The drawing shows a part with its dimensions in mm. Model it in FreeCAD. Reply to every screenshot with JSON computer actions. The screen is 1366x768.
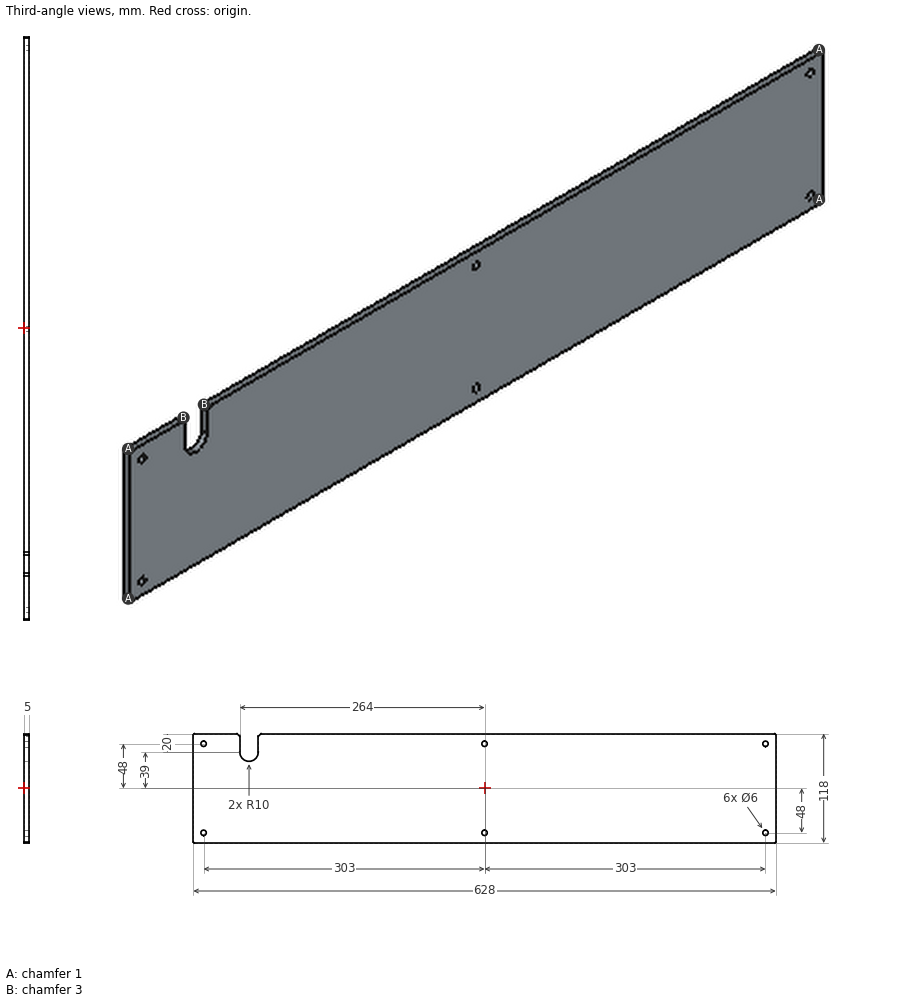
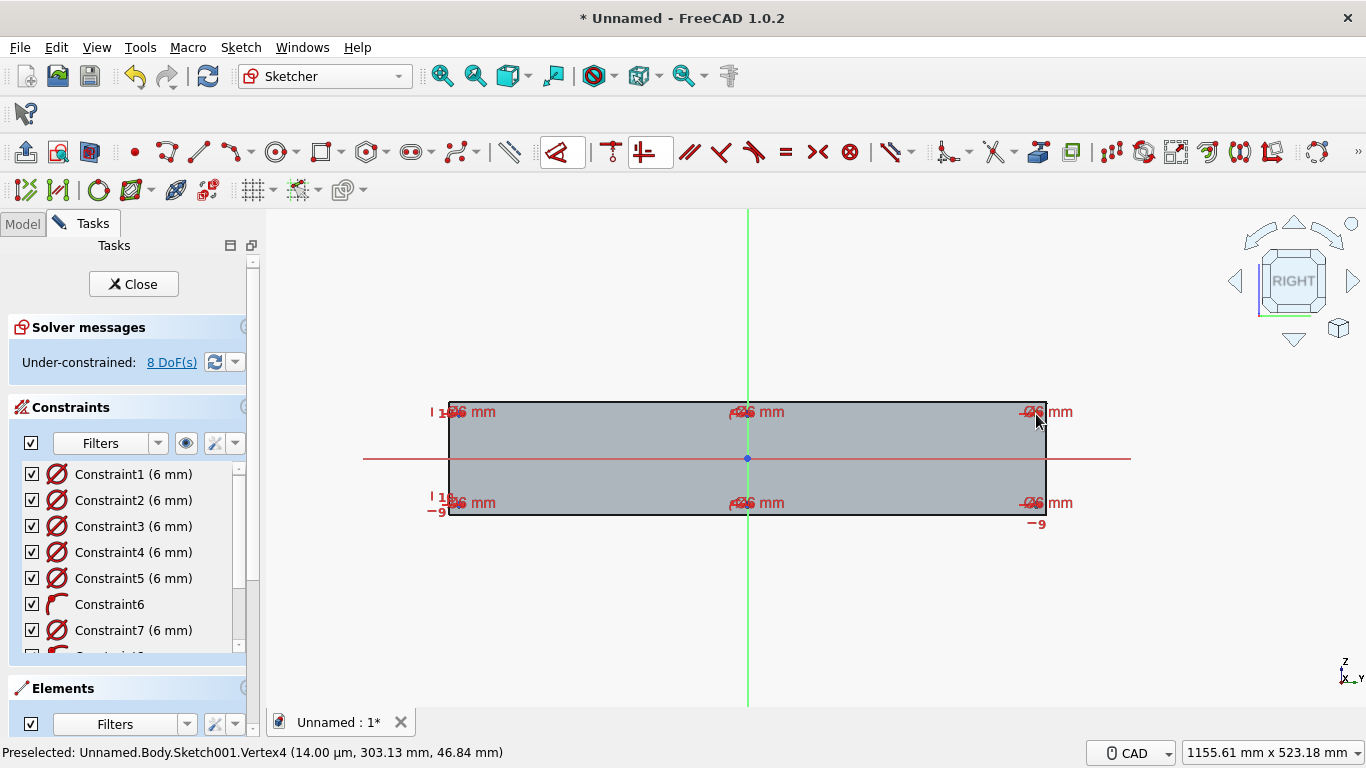
{"action": "left_click", "coordinate": [668, 152]}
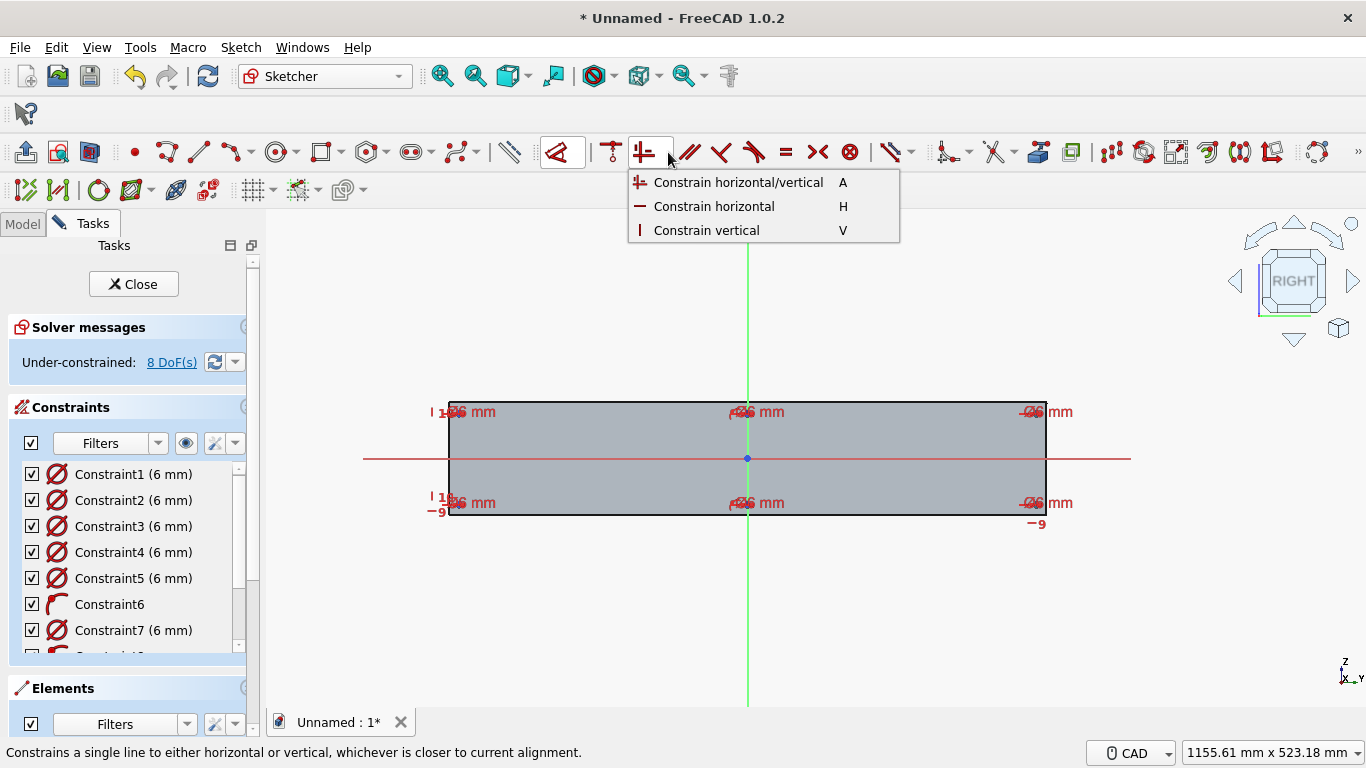
{"action": "left_click", "coordinate": [764, 230]}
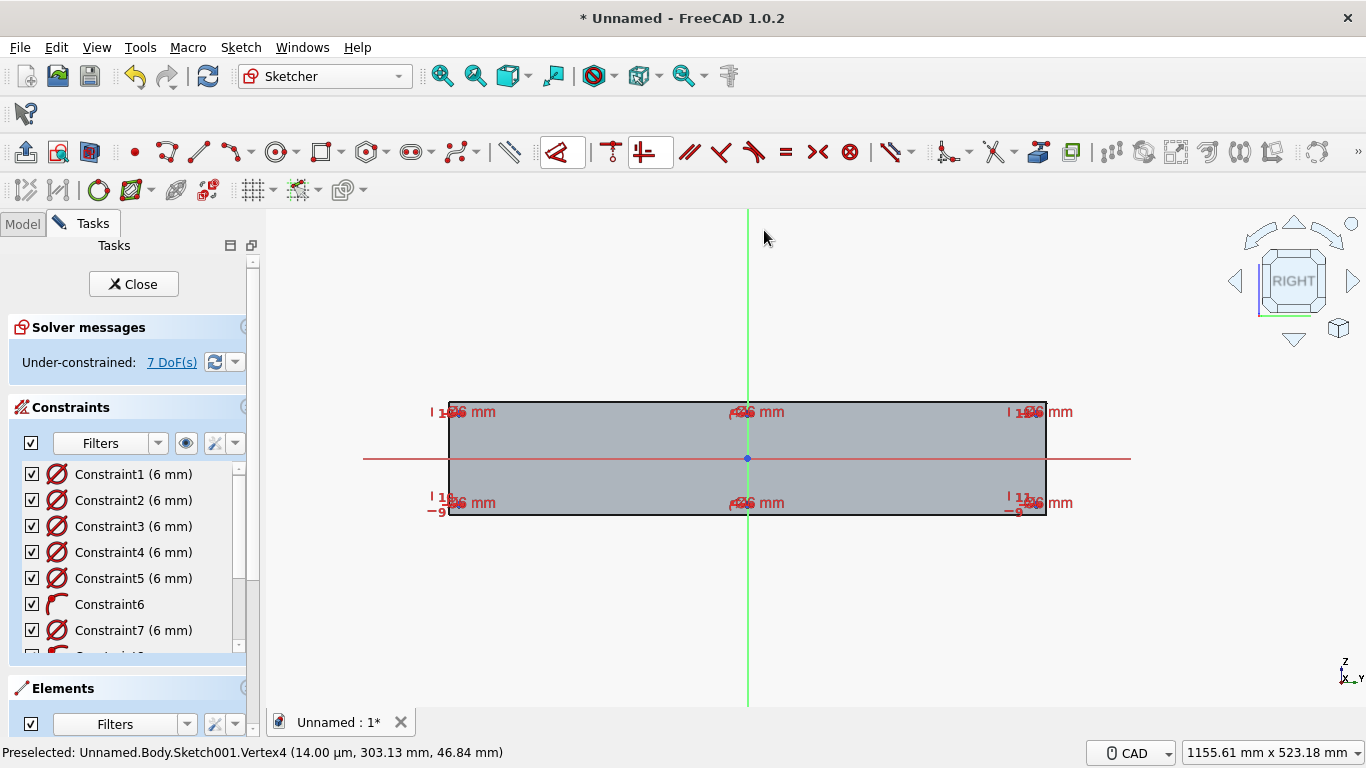
{"action": "left_click", "coordinate": [459, 414]}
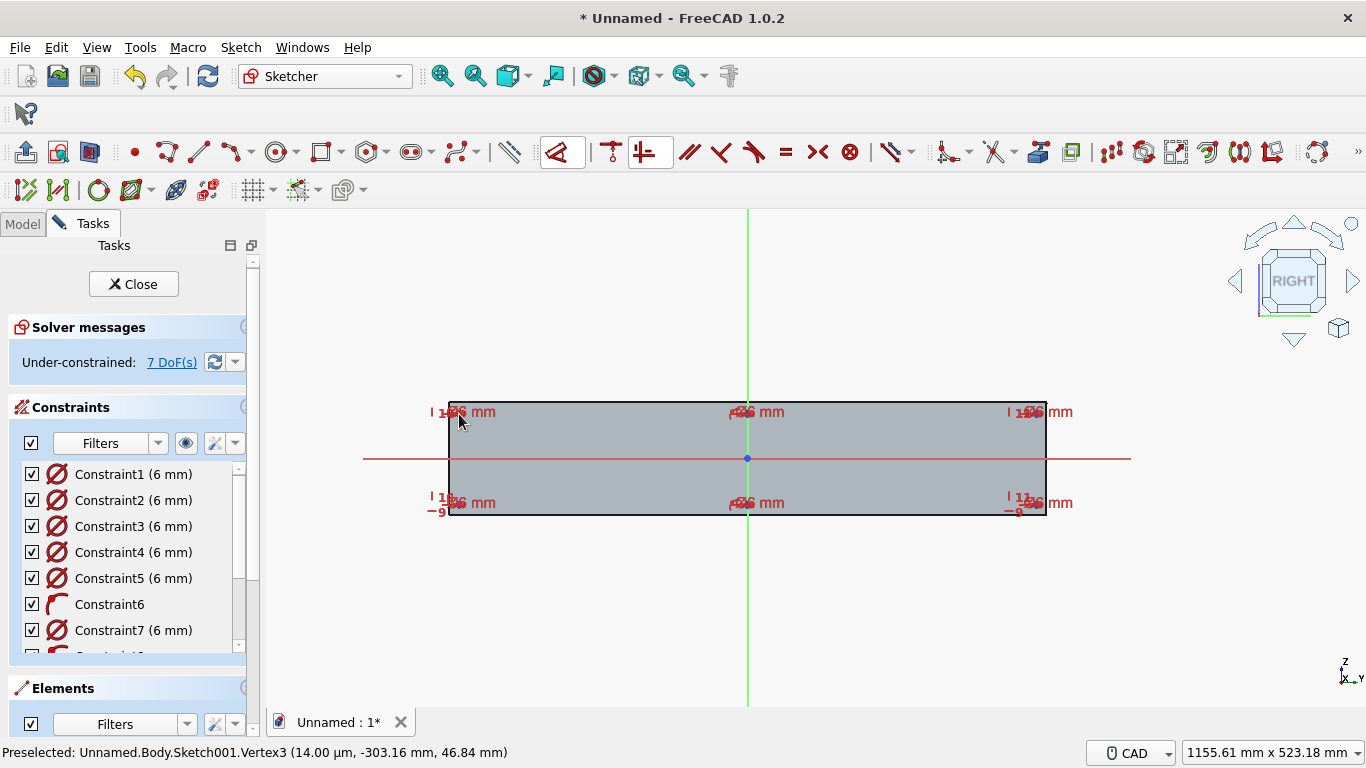
{"action": "left_click", "coordinate": [1036, 414]}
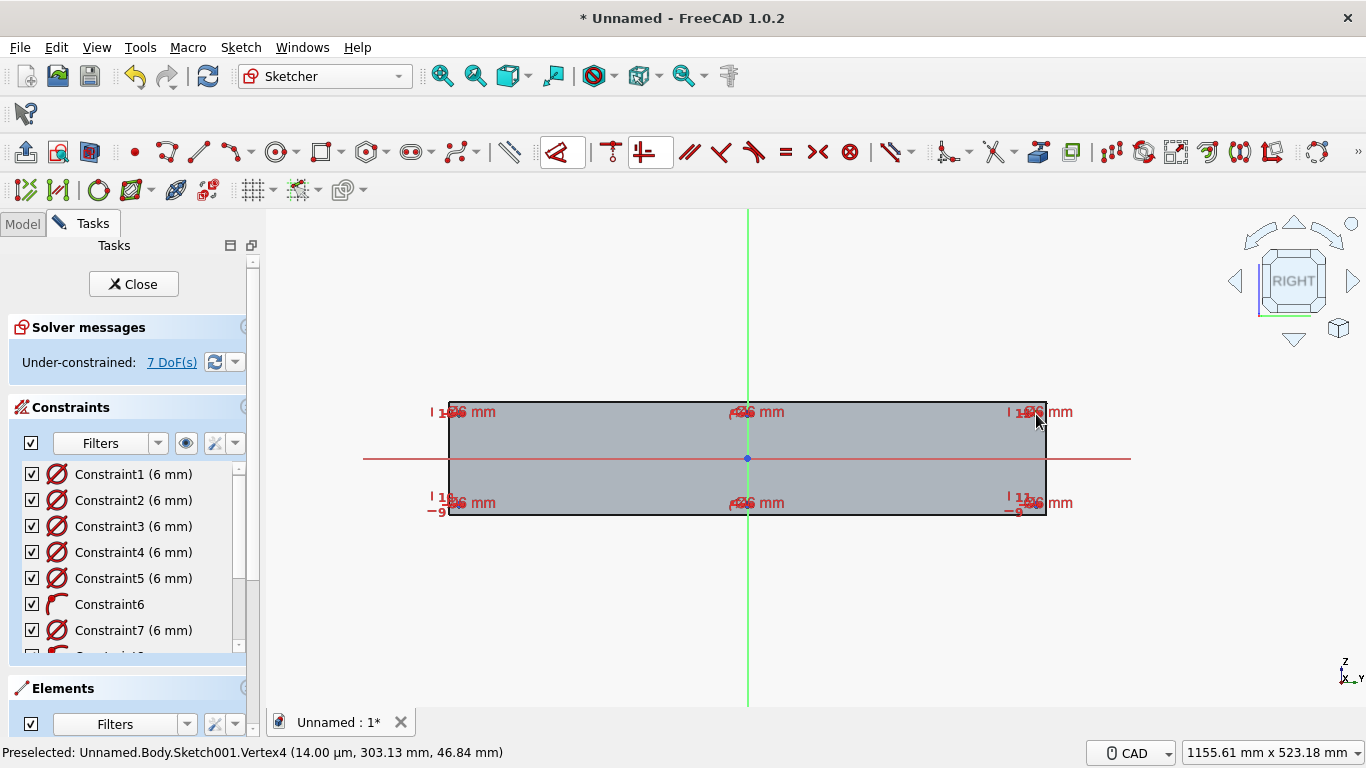
{"action": "key", "text": "h"}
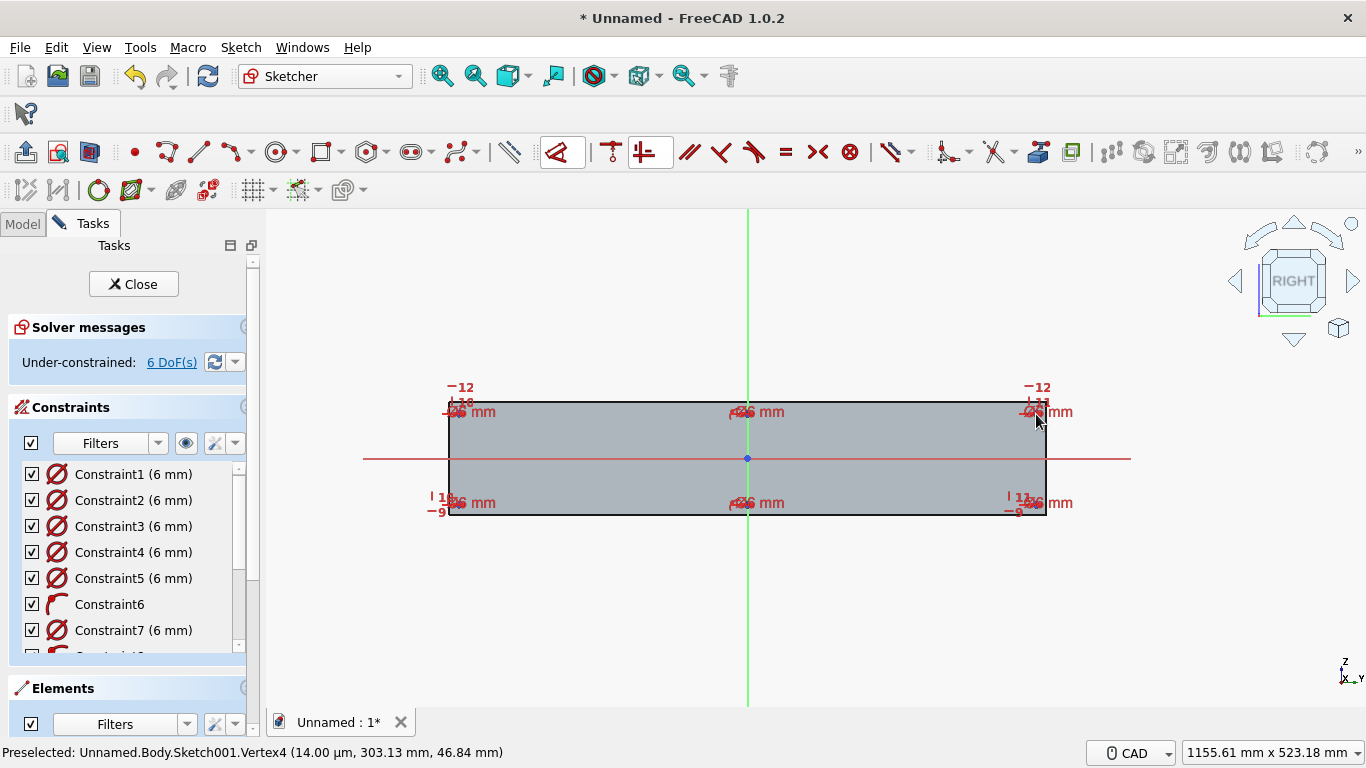
{"action": "left_click", "coordinate": [459, 414]}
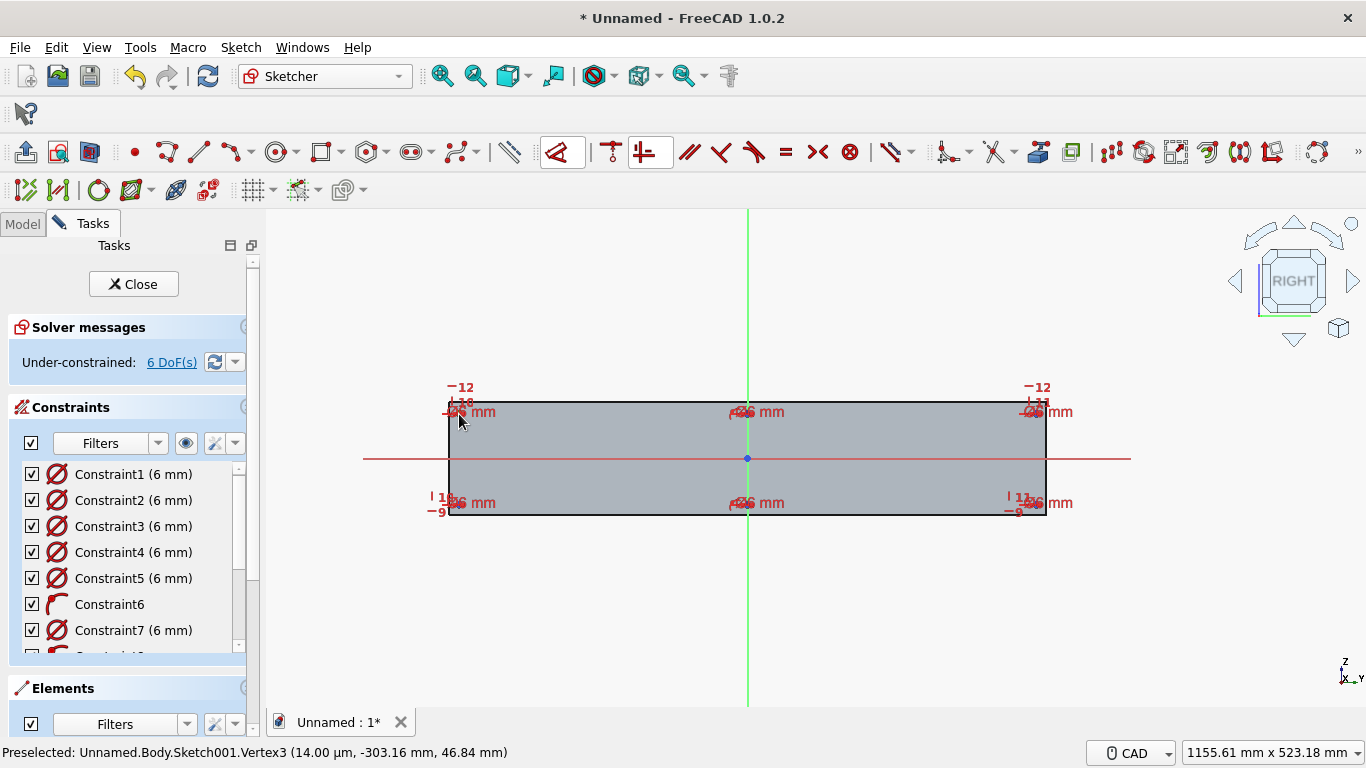
{"action": "left_click", "coordinate": [748, 414]}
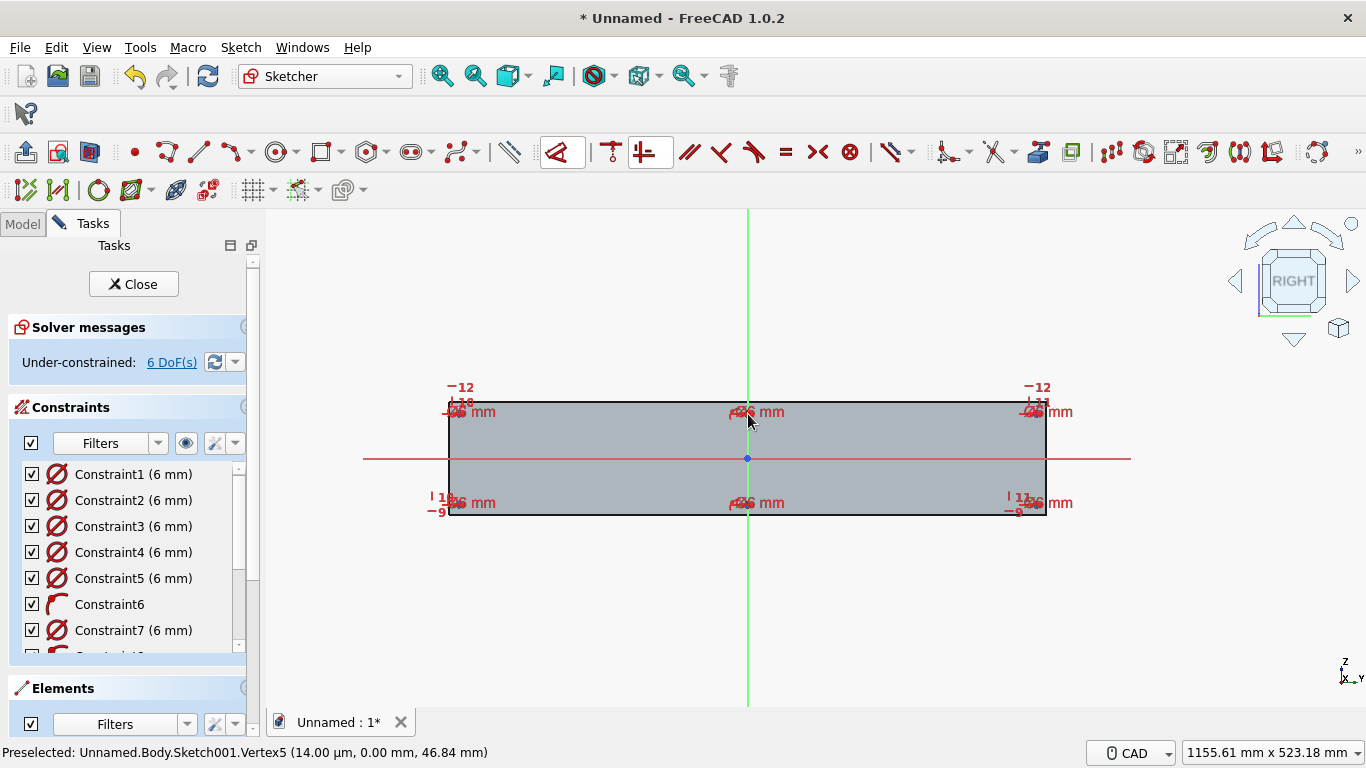
{"action": "key", "text": "h"}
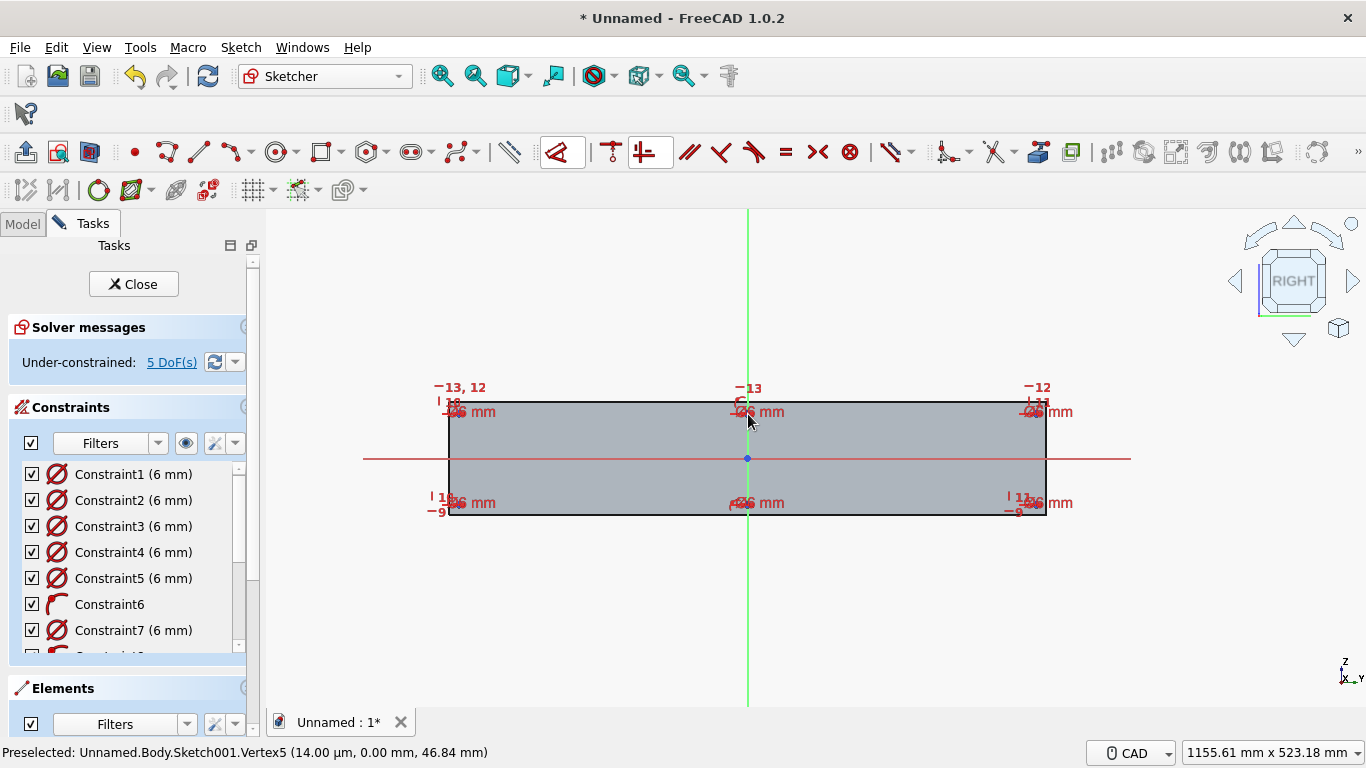
{"action": "left_click", "coordinate": [1036, 505]}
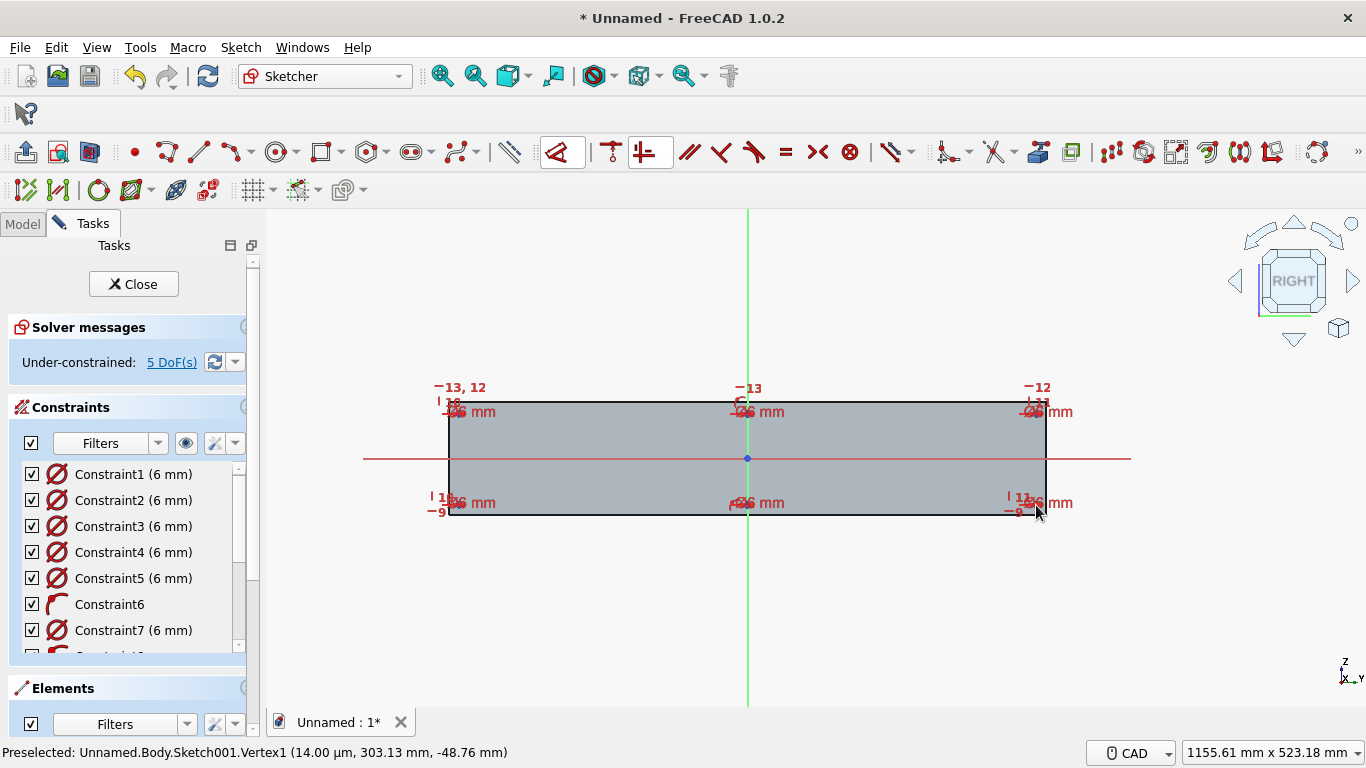
{"action": "left_click", "coordinate": [748, 505]}